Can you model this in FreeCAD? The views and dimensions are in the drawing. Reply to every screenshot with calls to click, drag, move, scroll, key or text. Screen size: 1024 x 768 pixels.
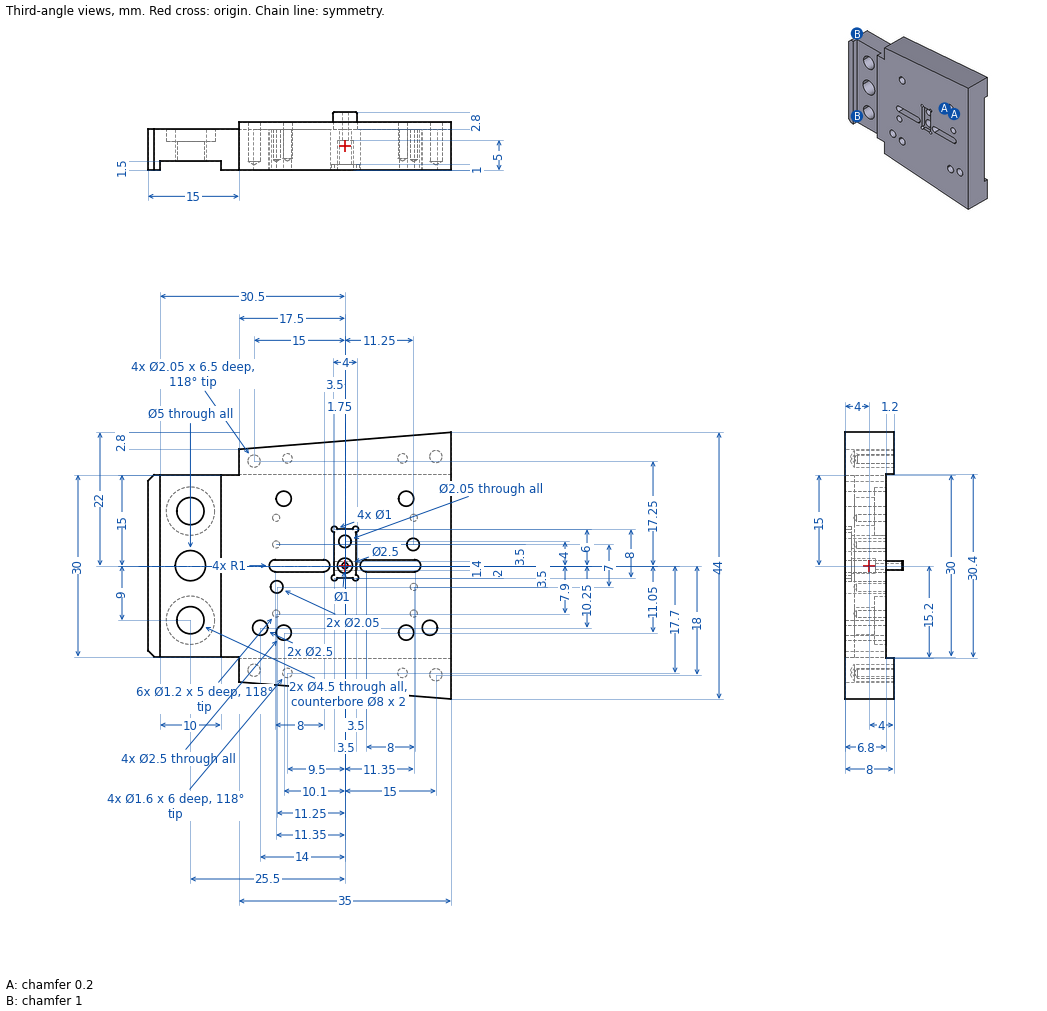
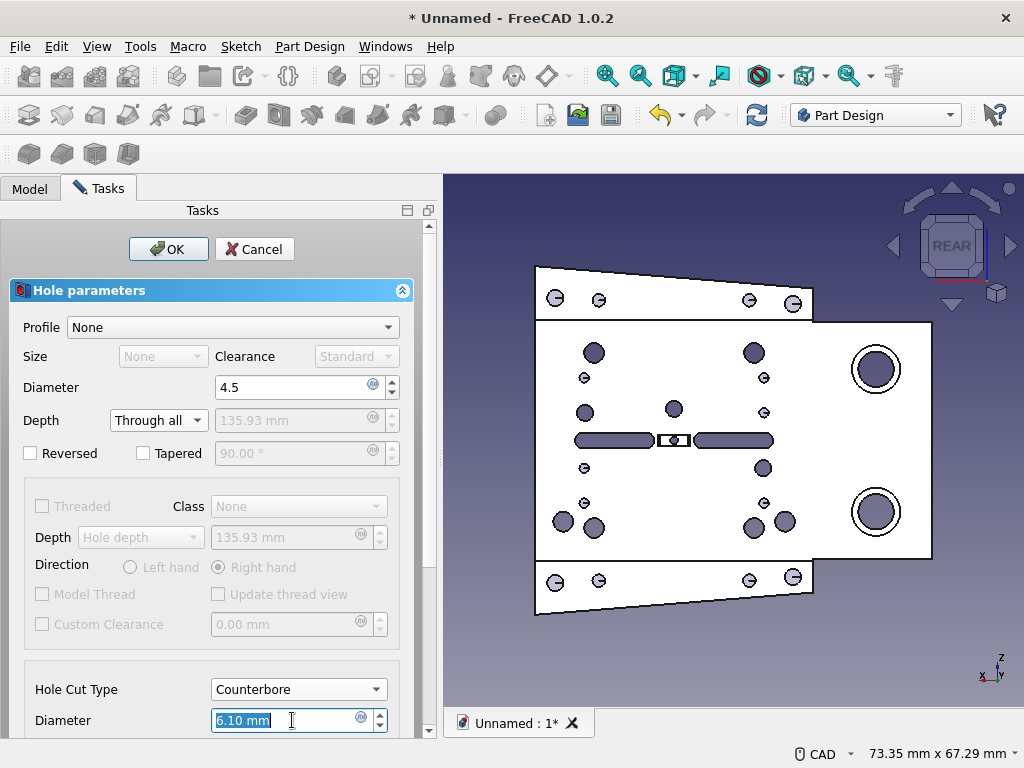
text(8)
key(Tab)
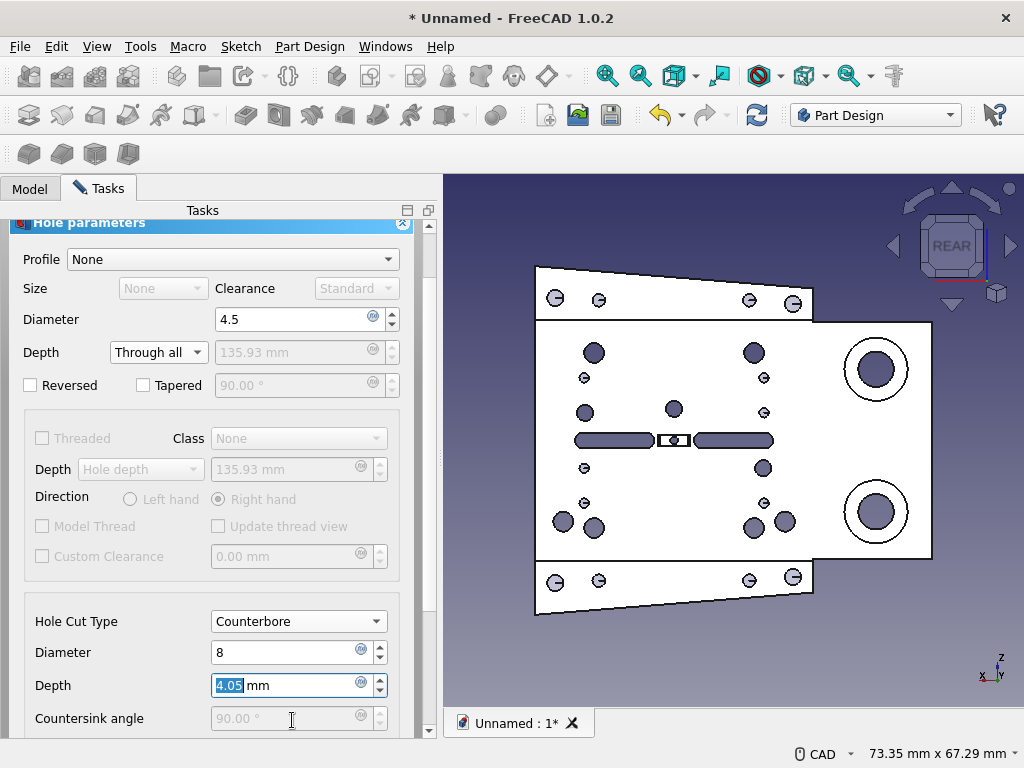
text(2)
key(Tab)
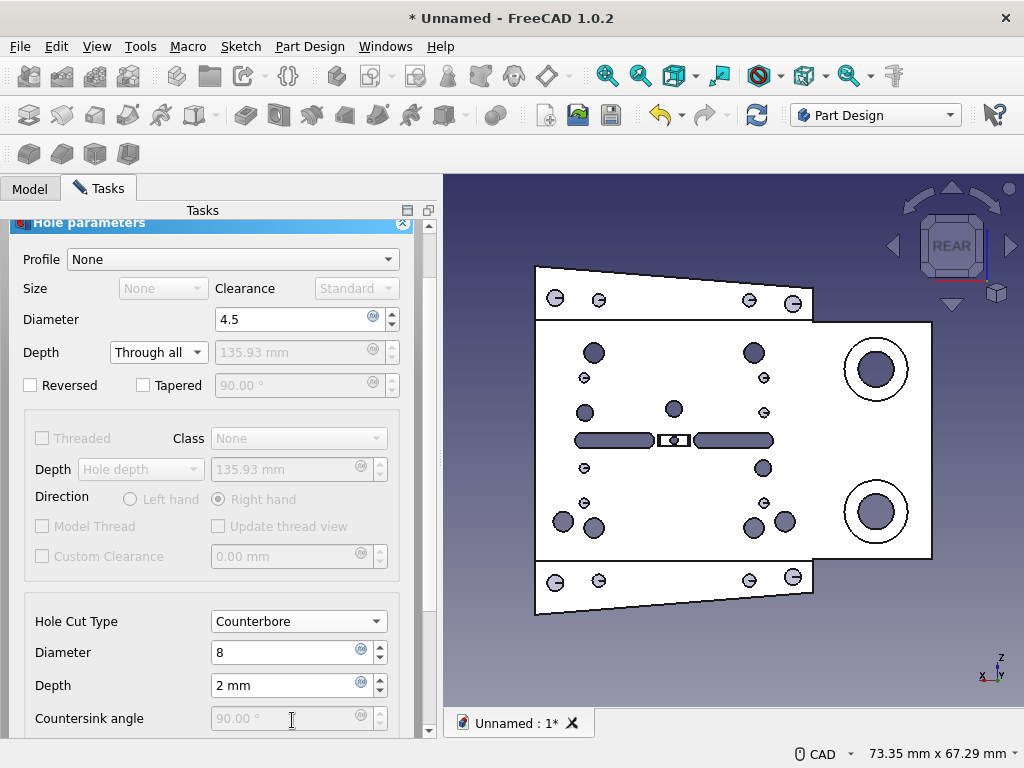
scroll(429, 479, up, 2)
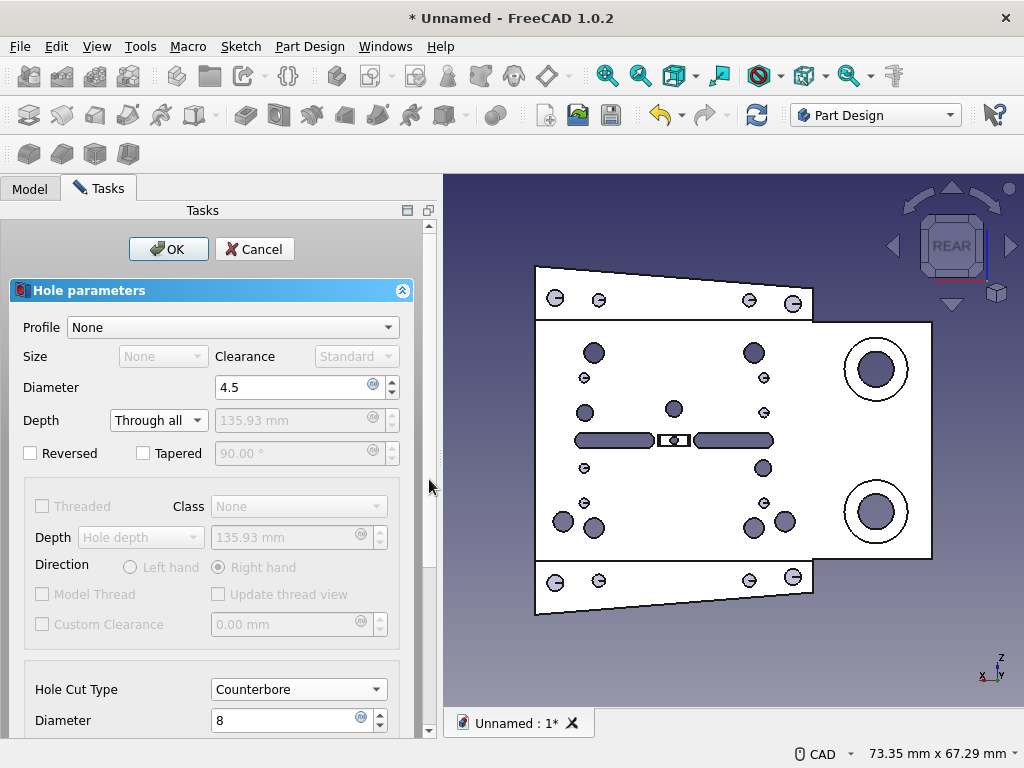
click(169, 249)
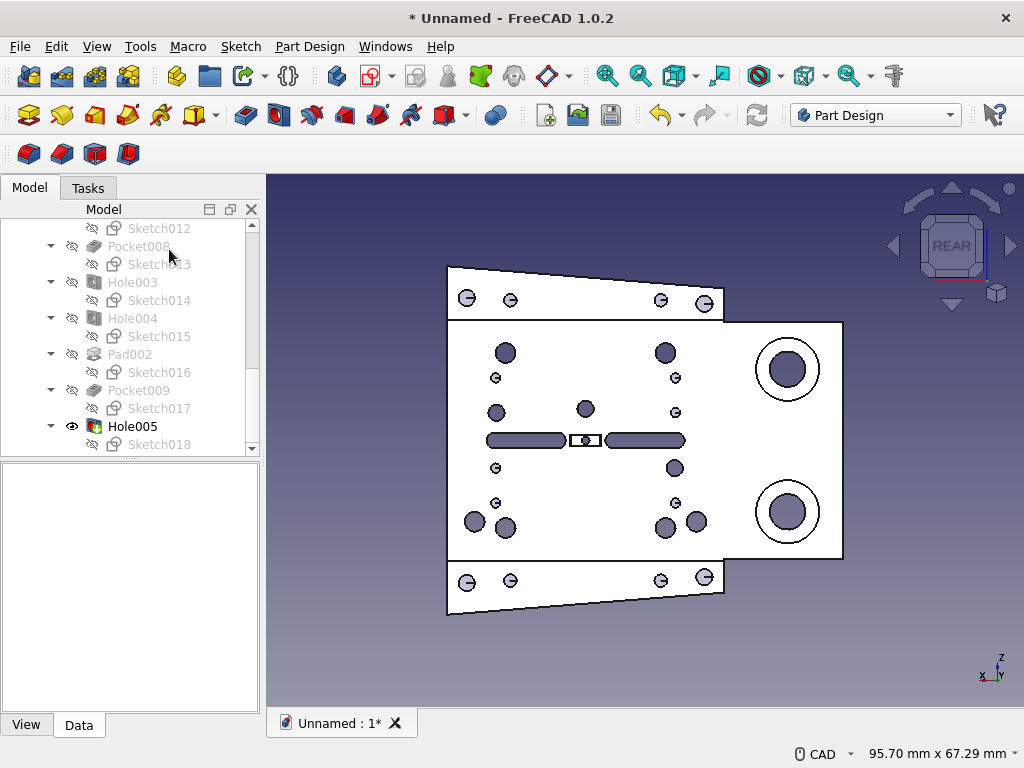
key(0)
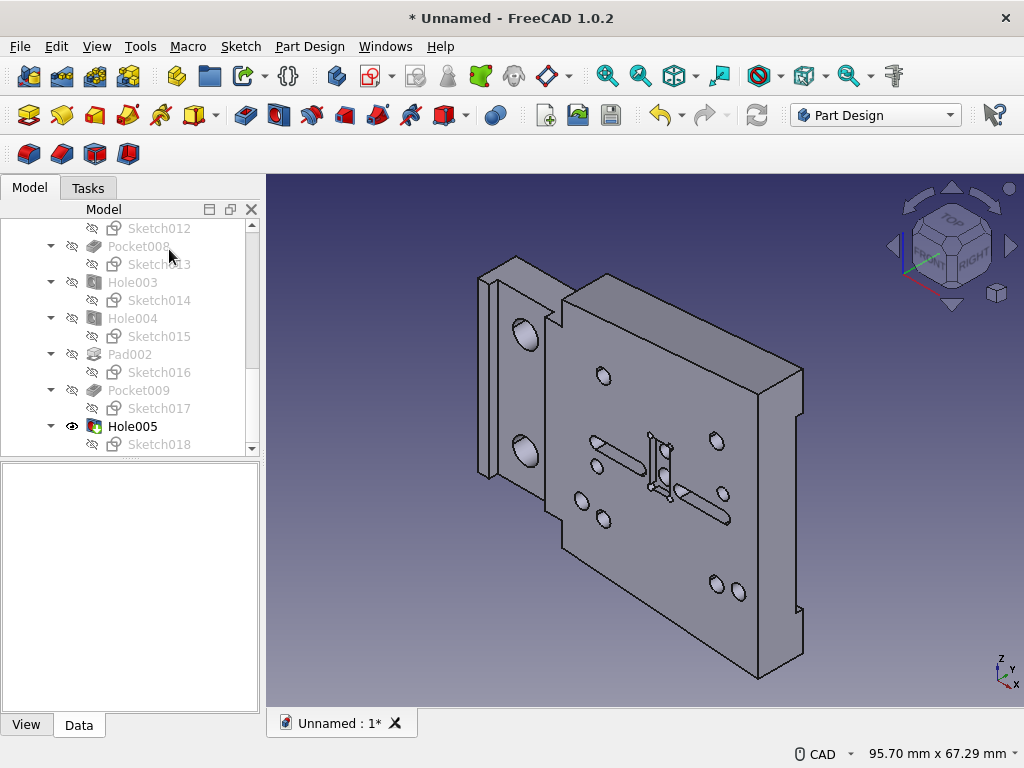
key(2)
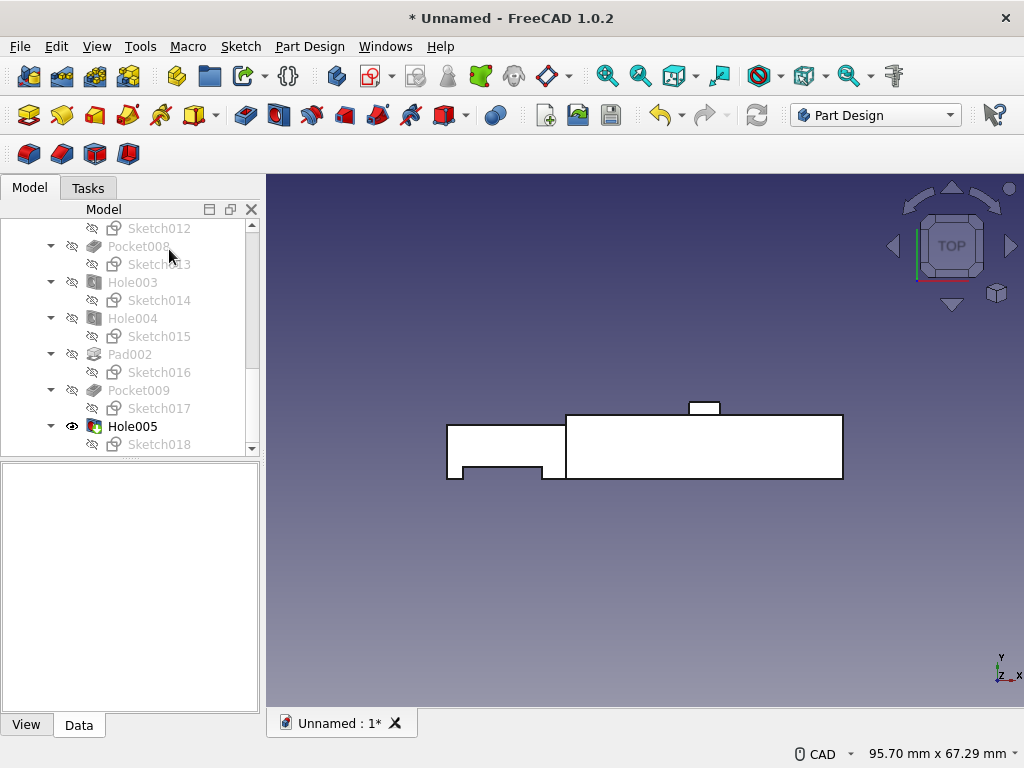
click(447, 451)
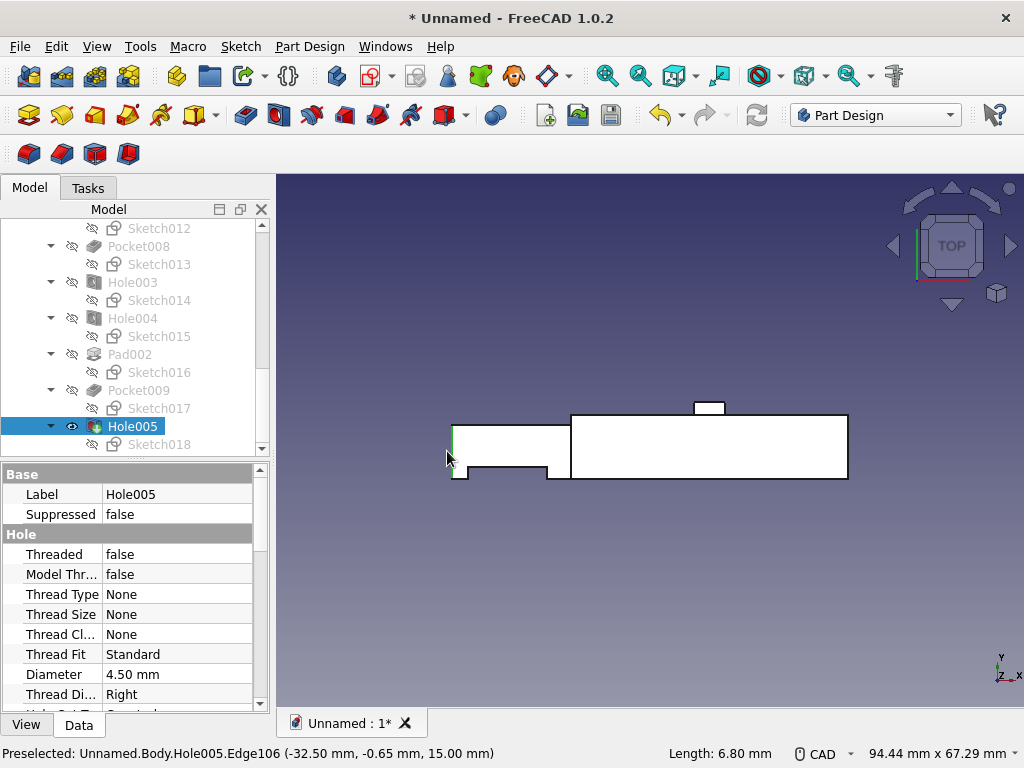
key(1)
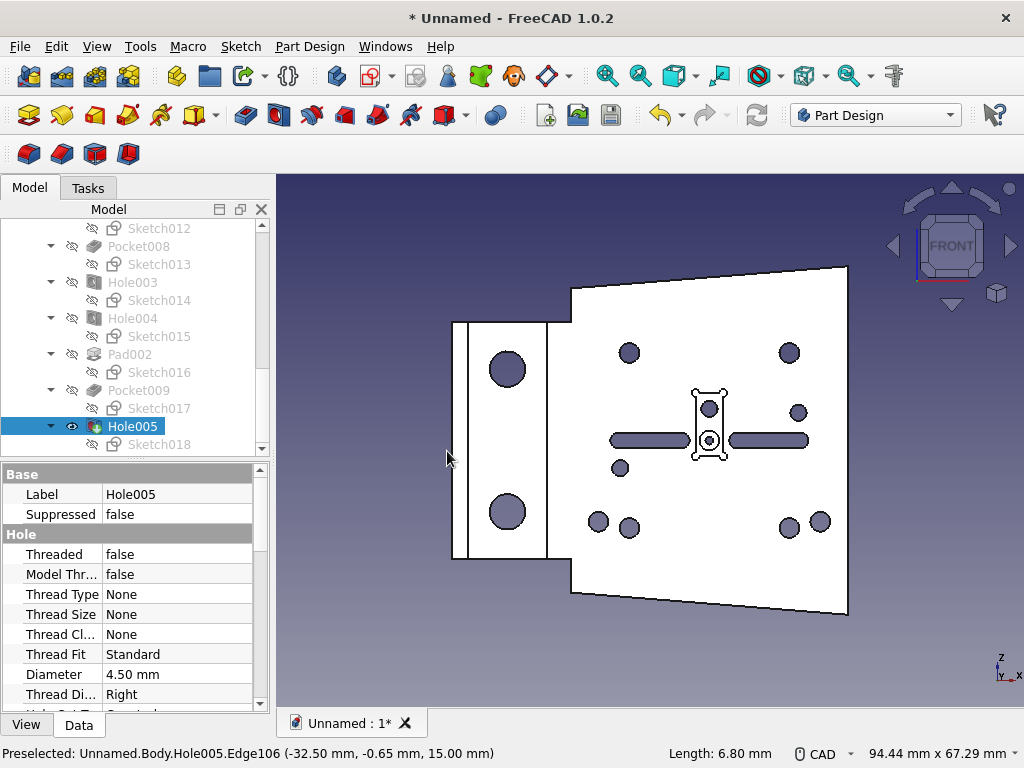
key(3)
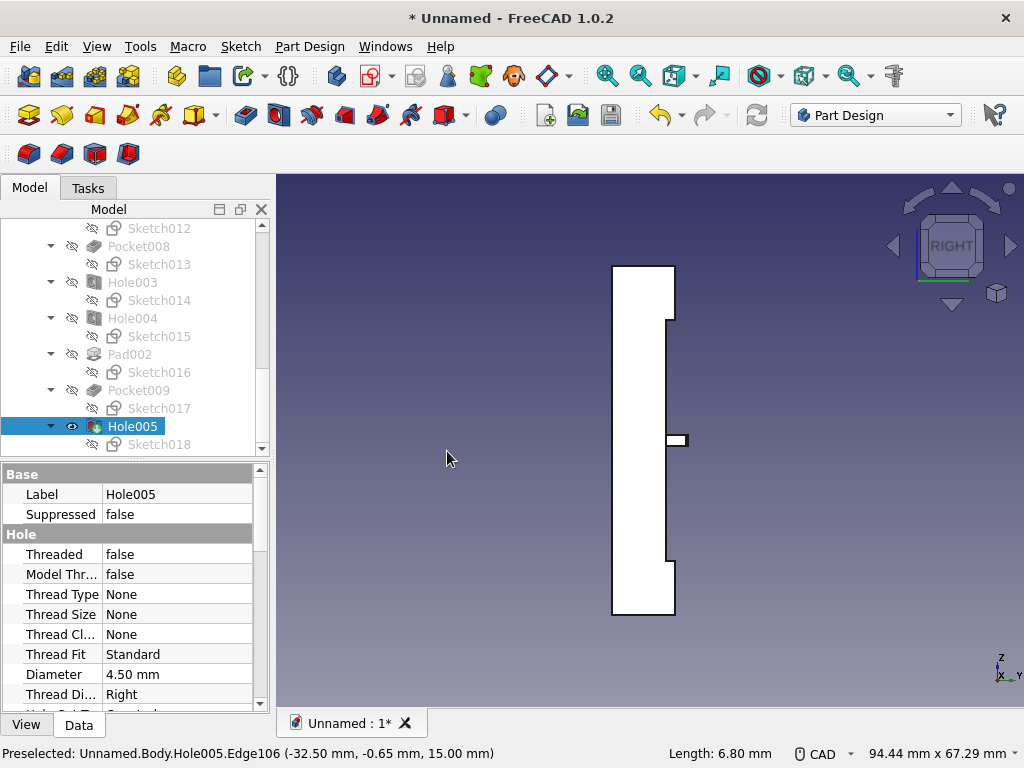
key(5)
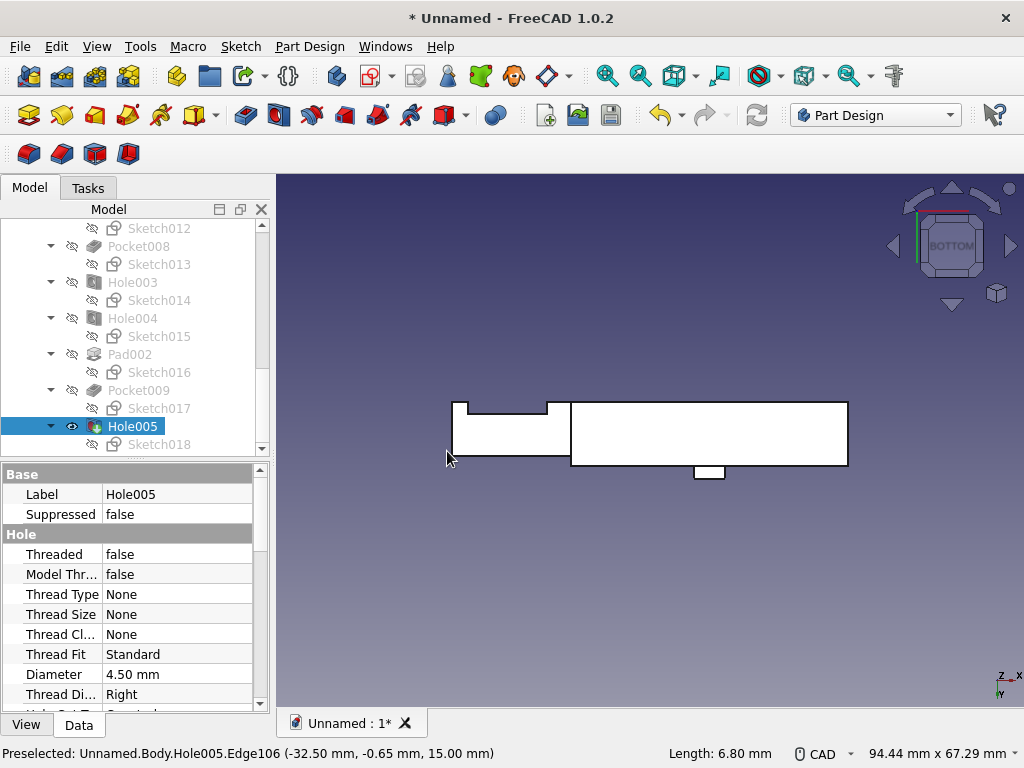
click(452, 428, ctrl)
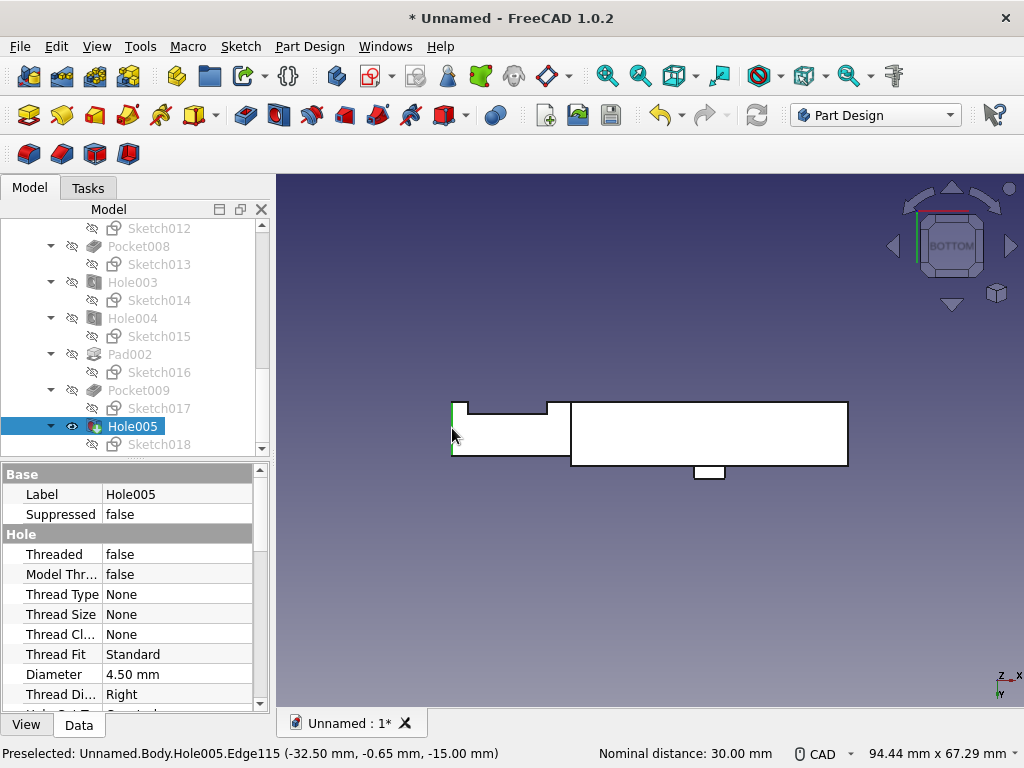
click(62, 154)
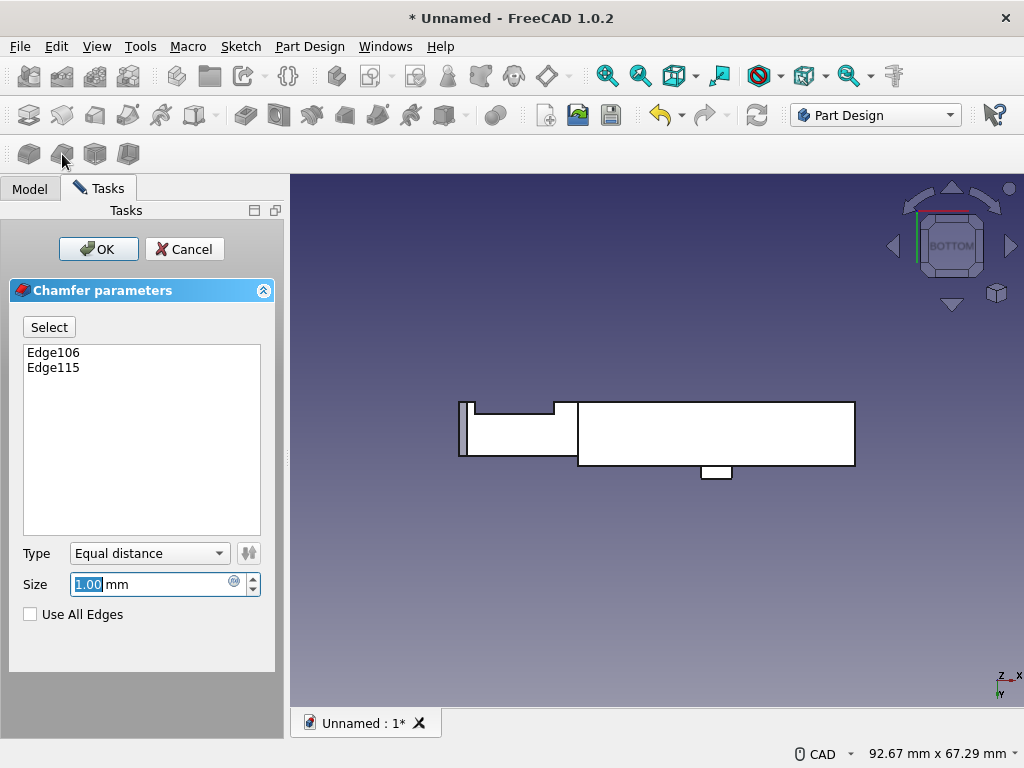
text(1)
key(Tab)